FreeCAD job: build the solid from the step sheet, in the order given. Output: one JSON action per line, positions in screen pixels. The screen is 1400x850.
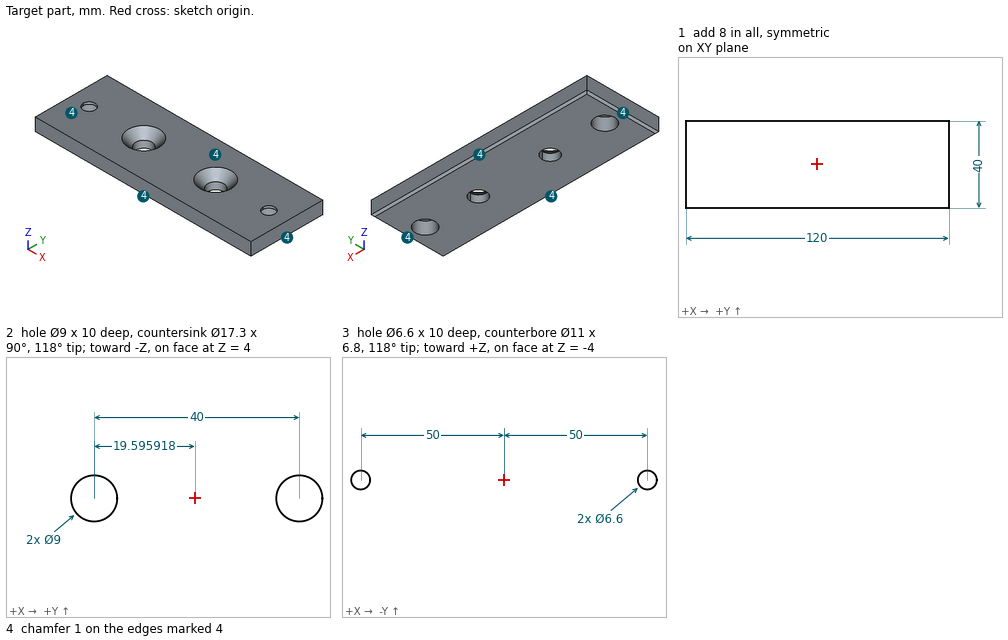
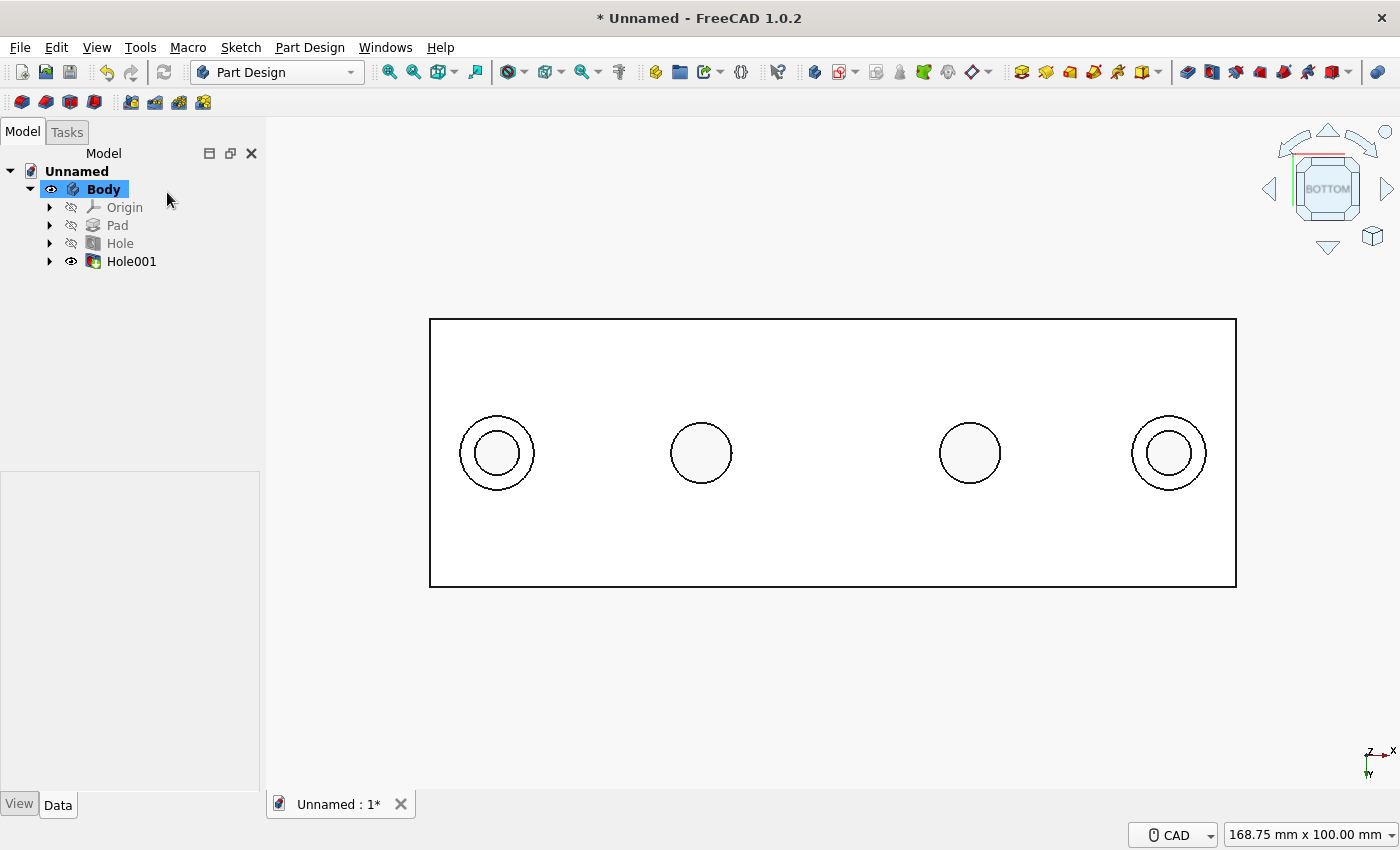
{"action": "left_click", "coordinate": [430, 452]}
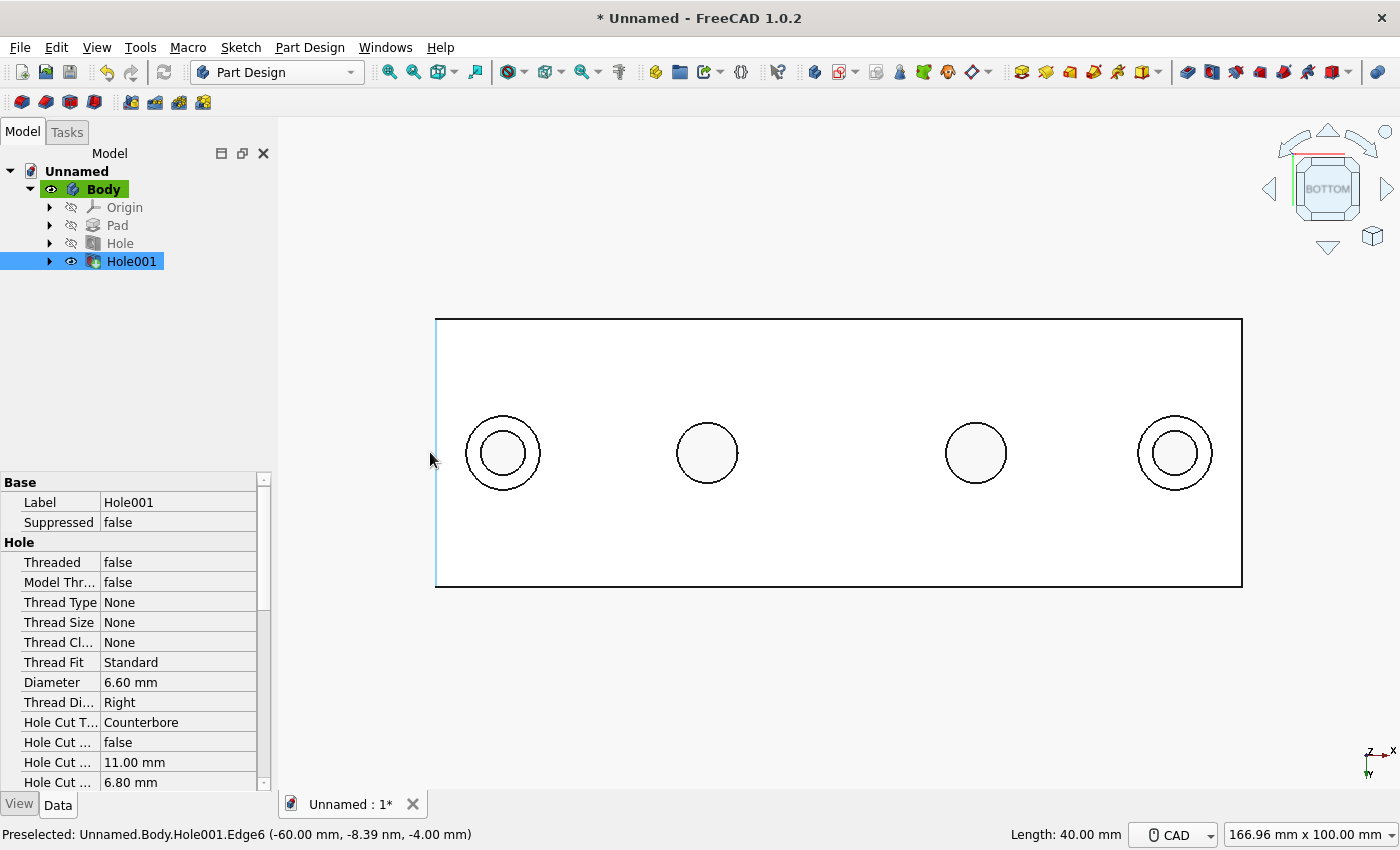
{"action": "left_click", "coordinate": [839, 586], "text": "ctrl"}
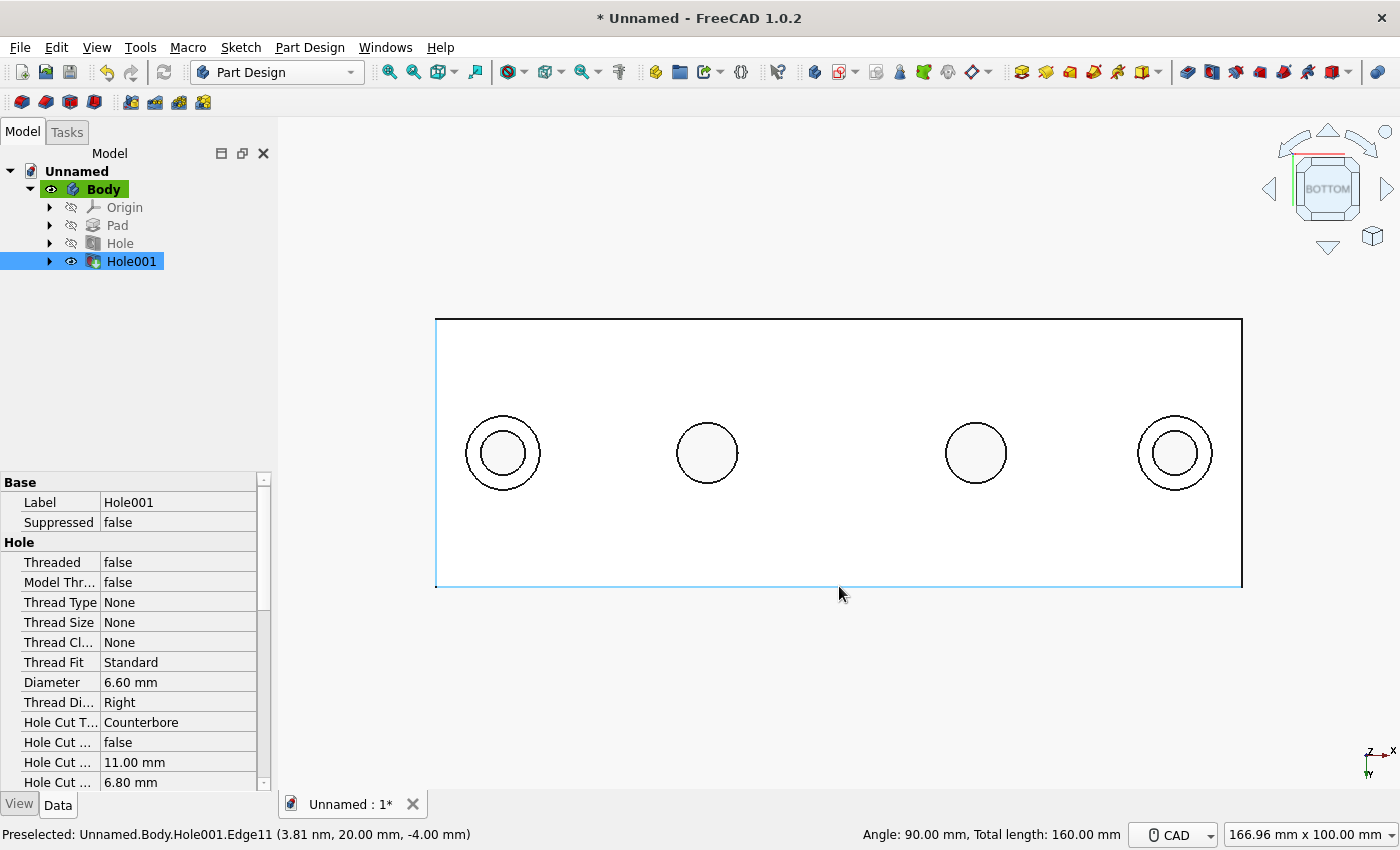
{"action": "left_click", "coordinate": [1242, 452], "text": "ctrl"}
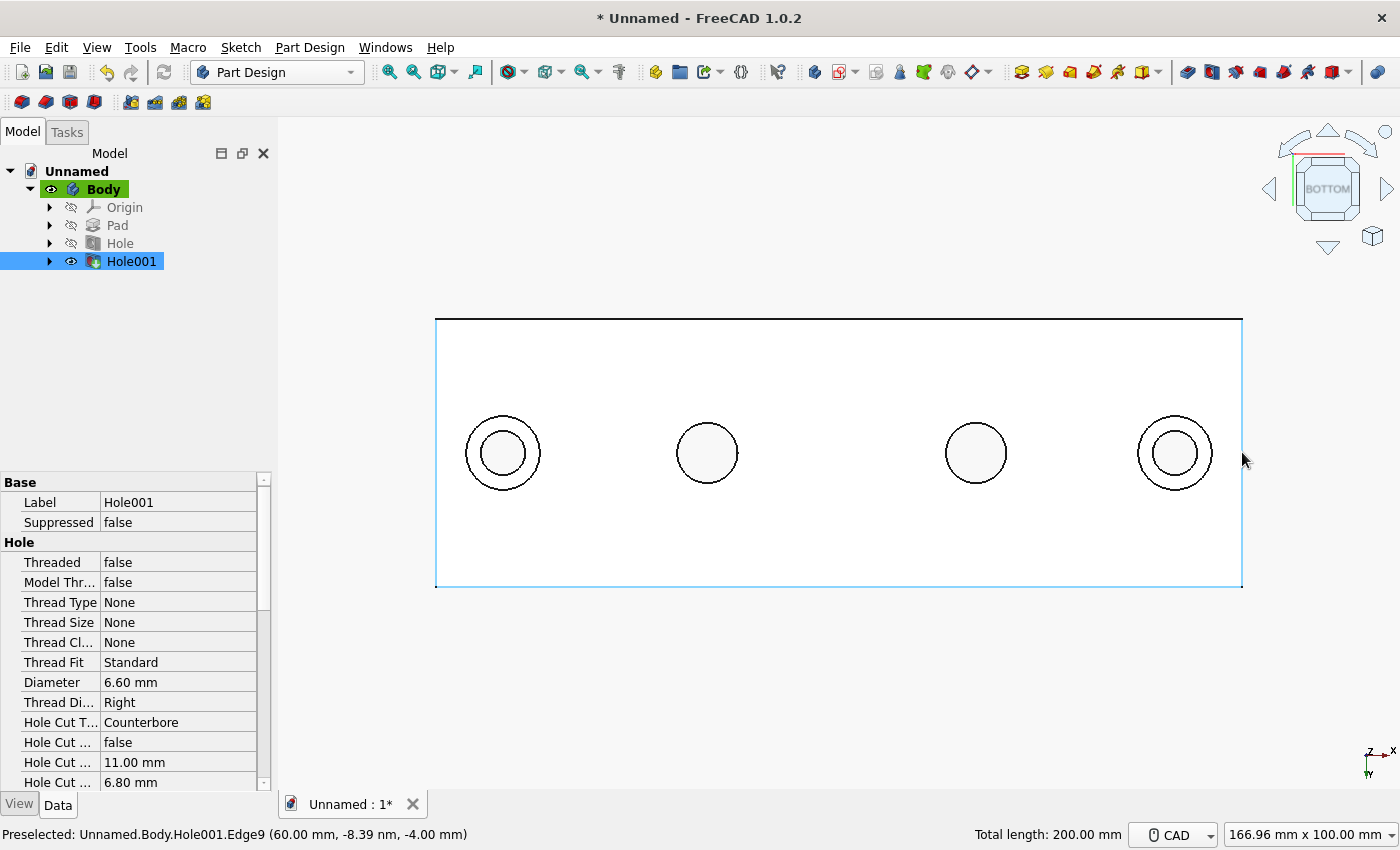
{"action": "key", "text": "0"}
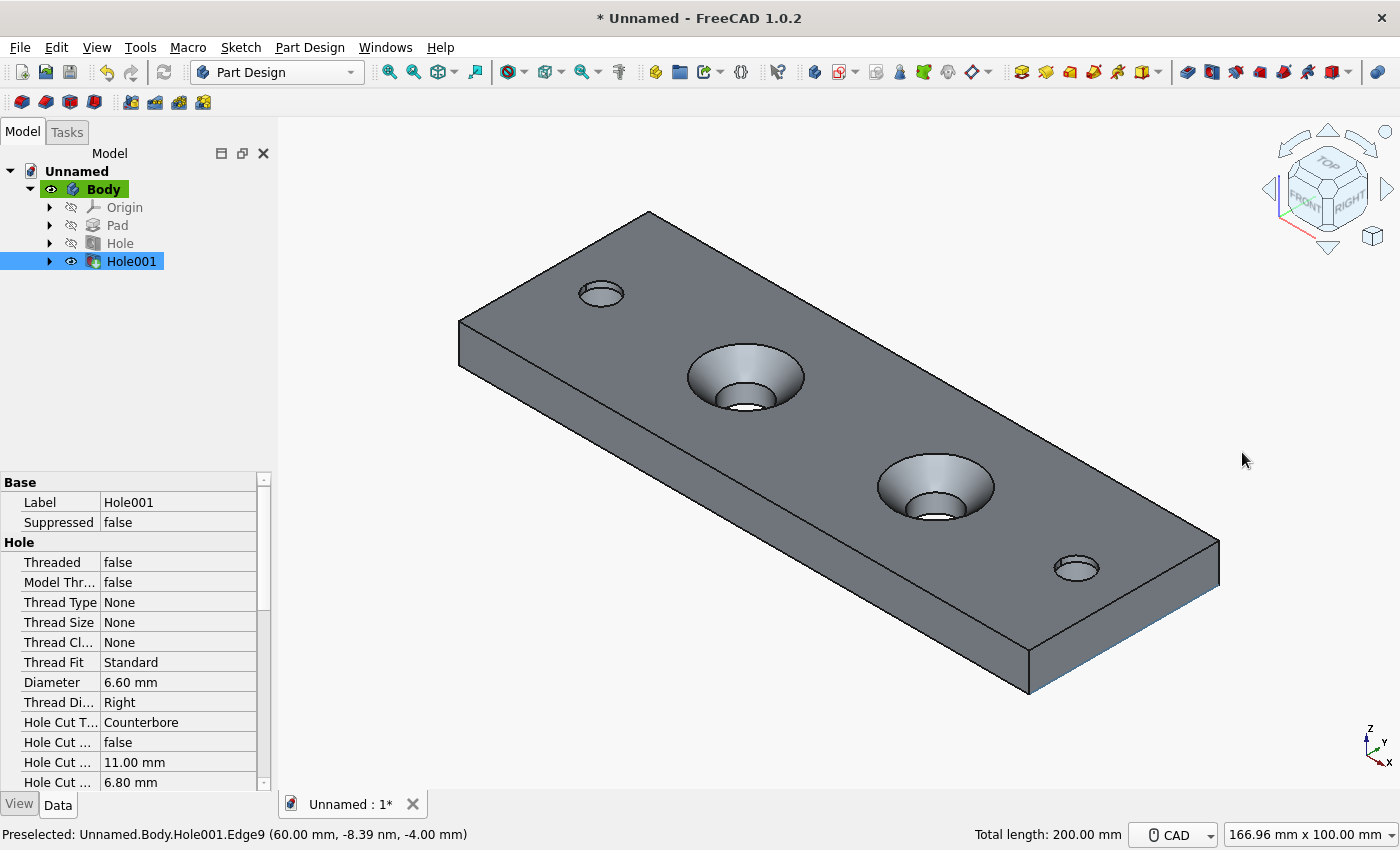
{"action": "key", "text": "2"}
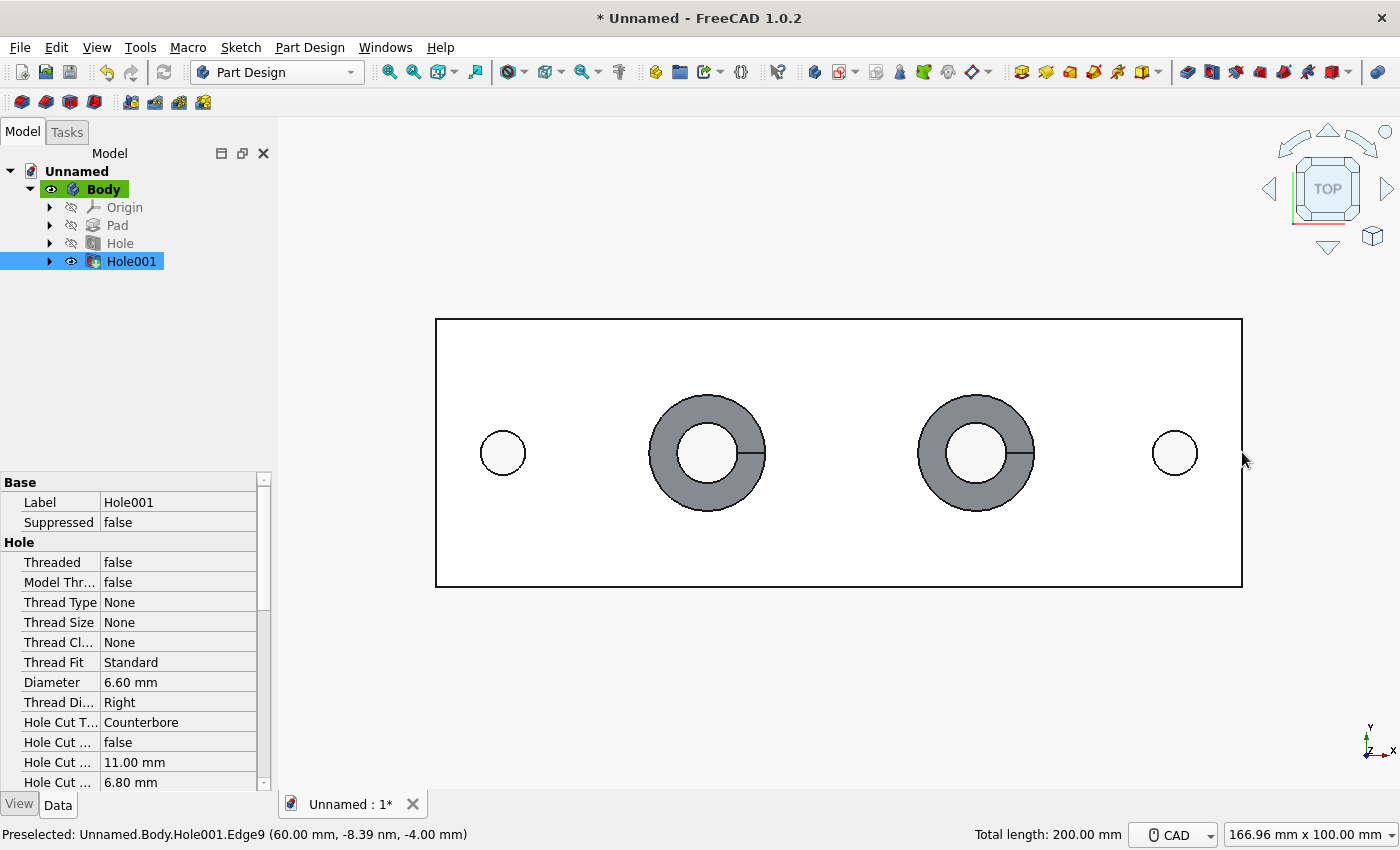
{"action": "key", "text": "1"}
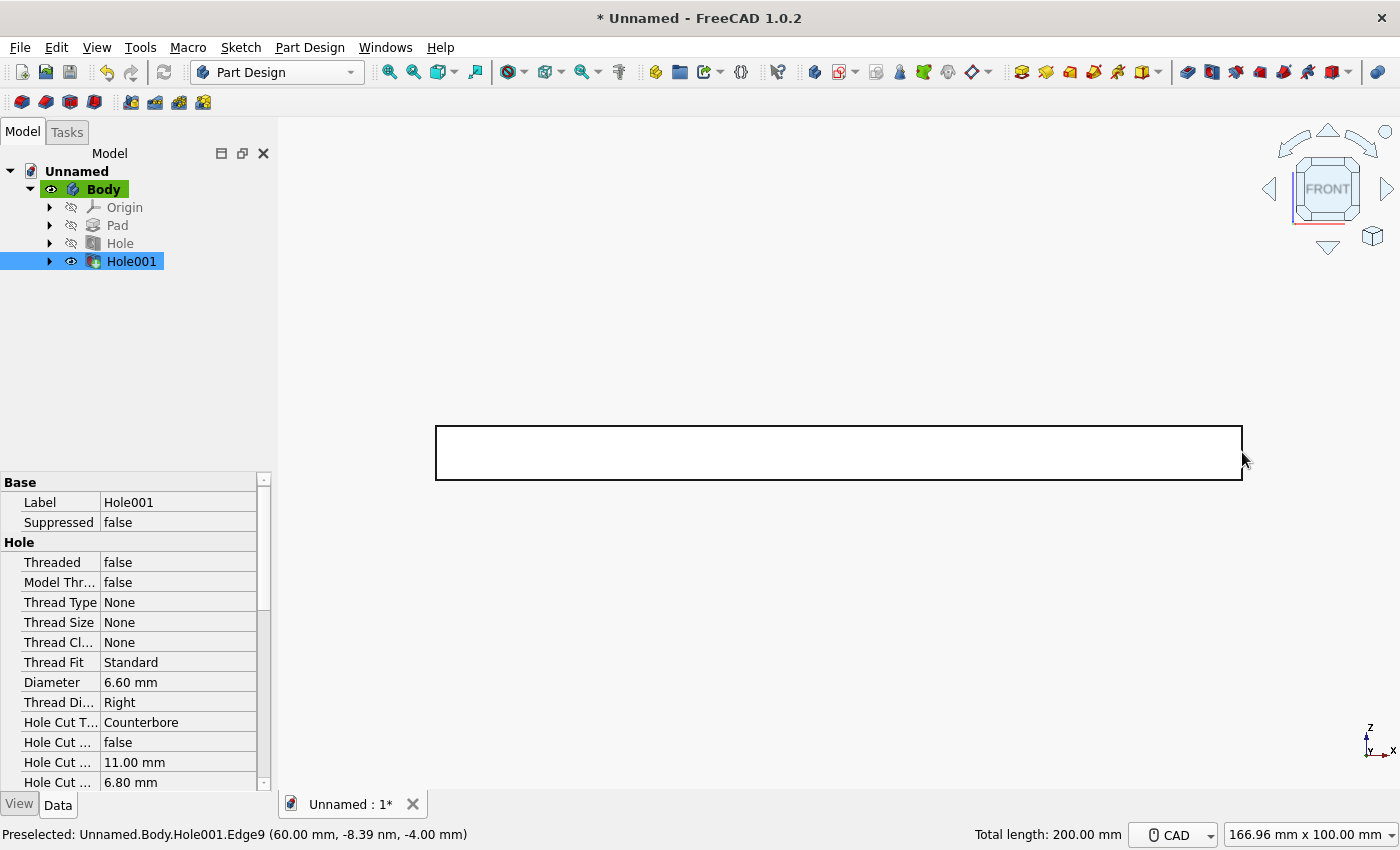
{"action": "left_click", "coordinate": [839, 479], "text": "ctrl"}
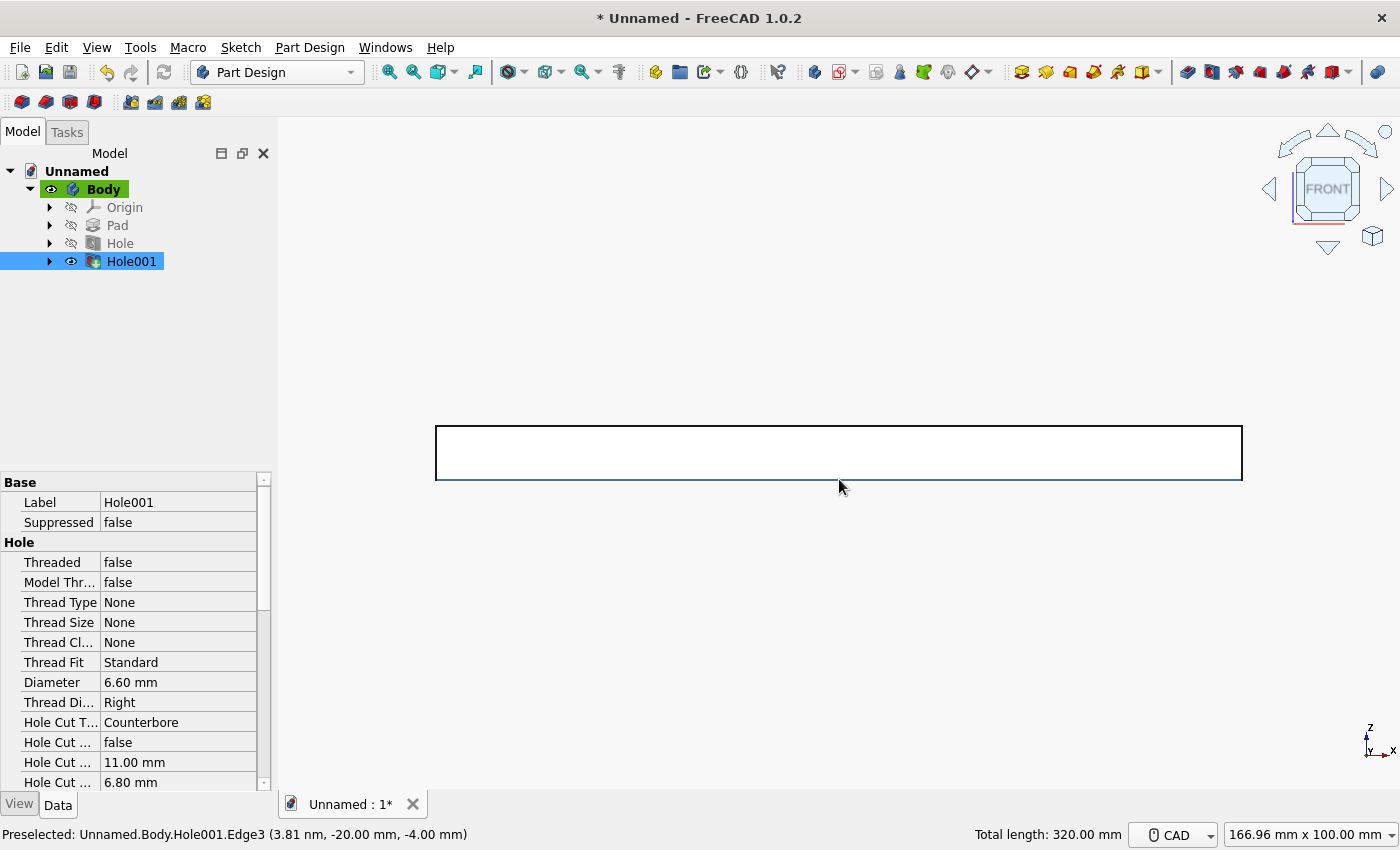
{"action": "left_click", "coordinate": [46, 102]}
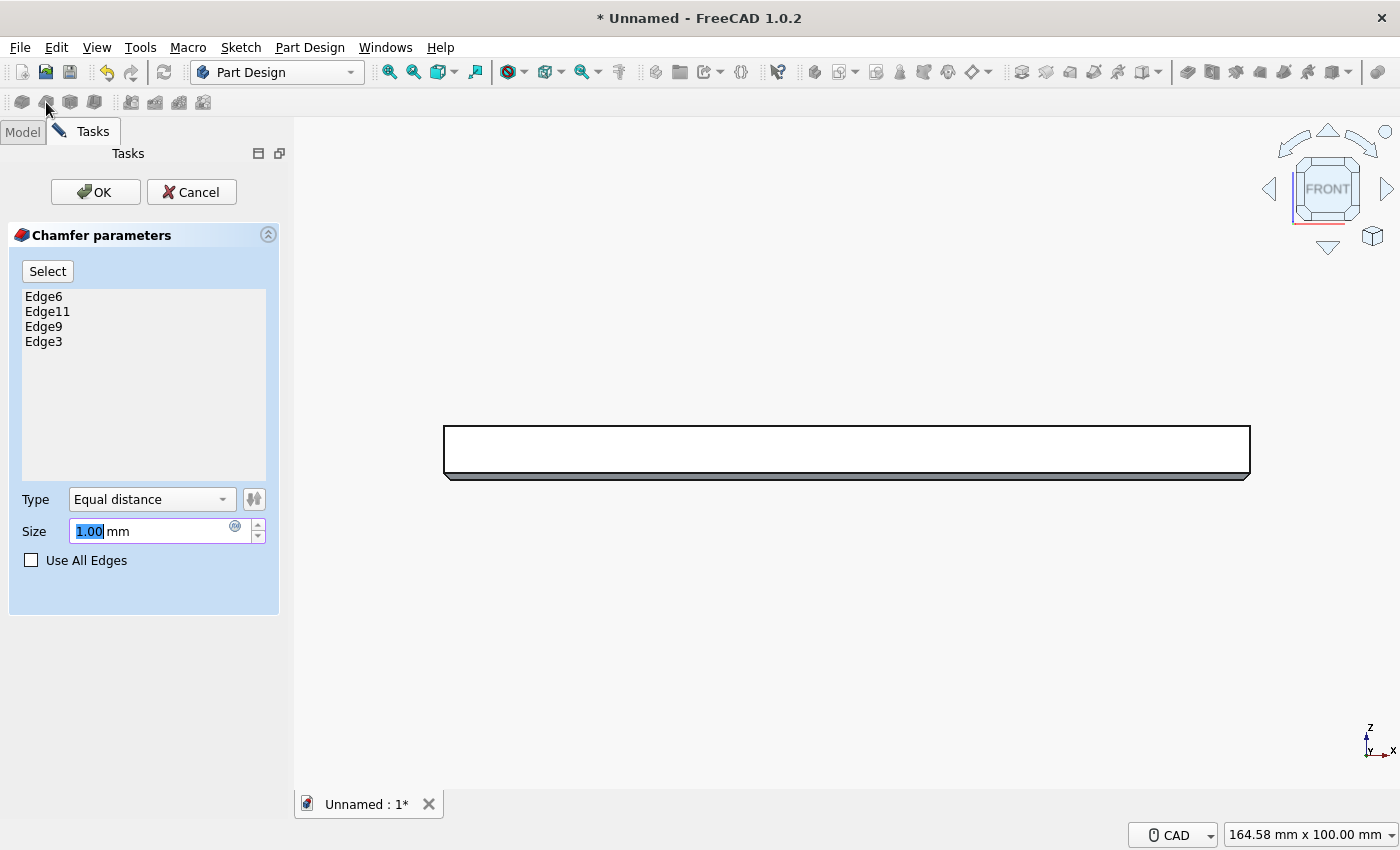
{"action": "type", "text": "1"}
{"action": "key", "text": "Tab"}